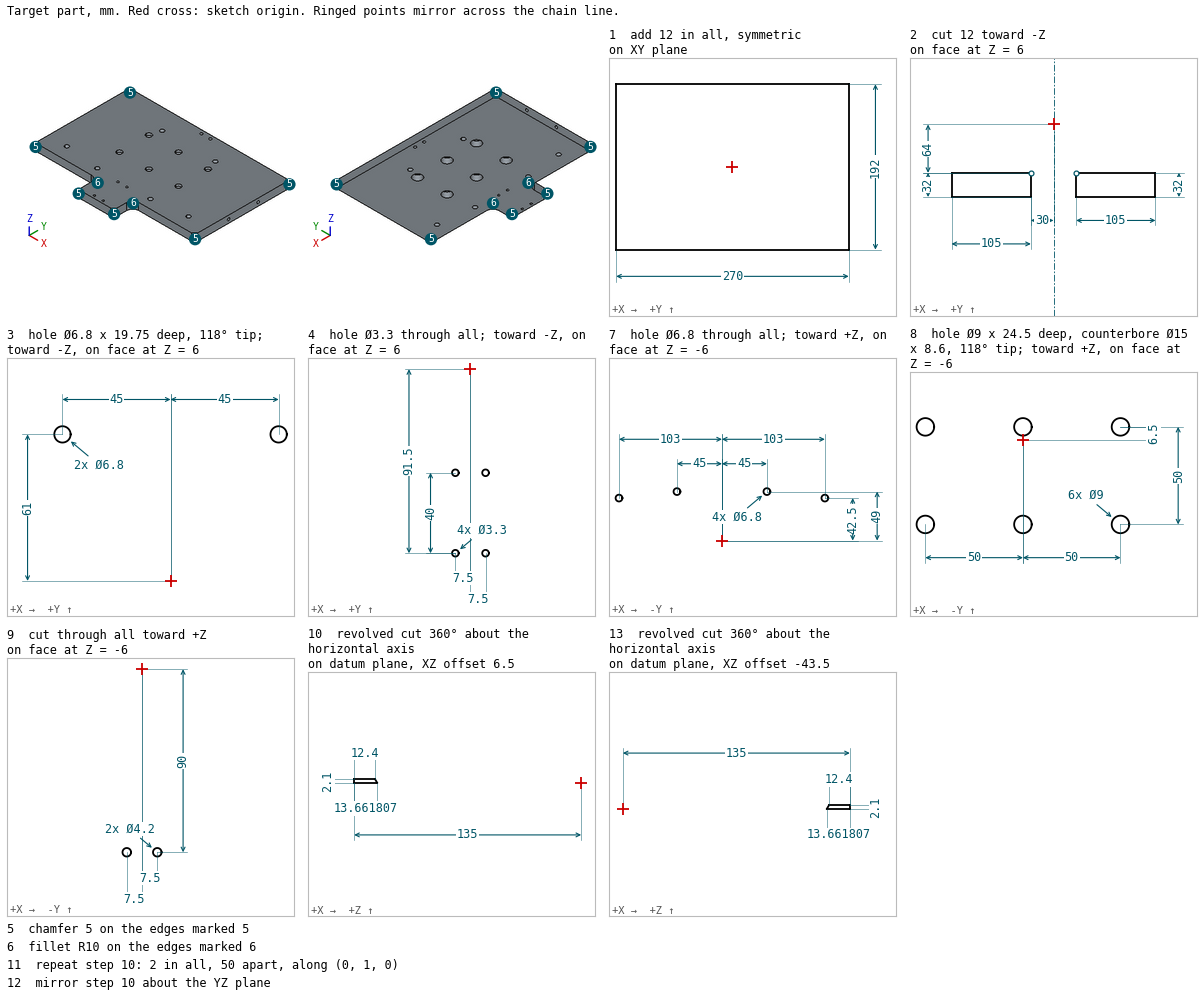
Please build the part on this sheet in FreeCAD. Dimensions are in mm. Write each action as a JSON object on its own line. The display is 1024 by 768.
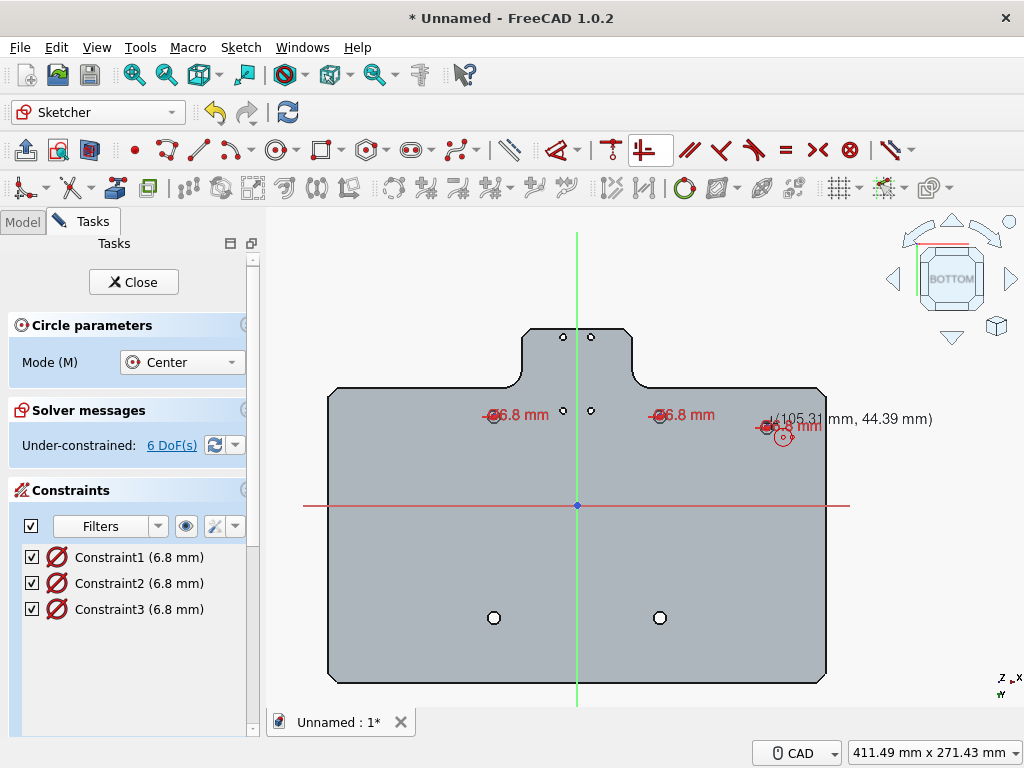
{"action": "scroll", "coordinate": [387, 427], "scroll_direction": "up", "scroll_amount": 7}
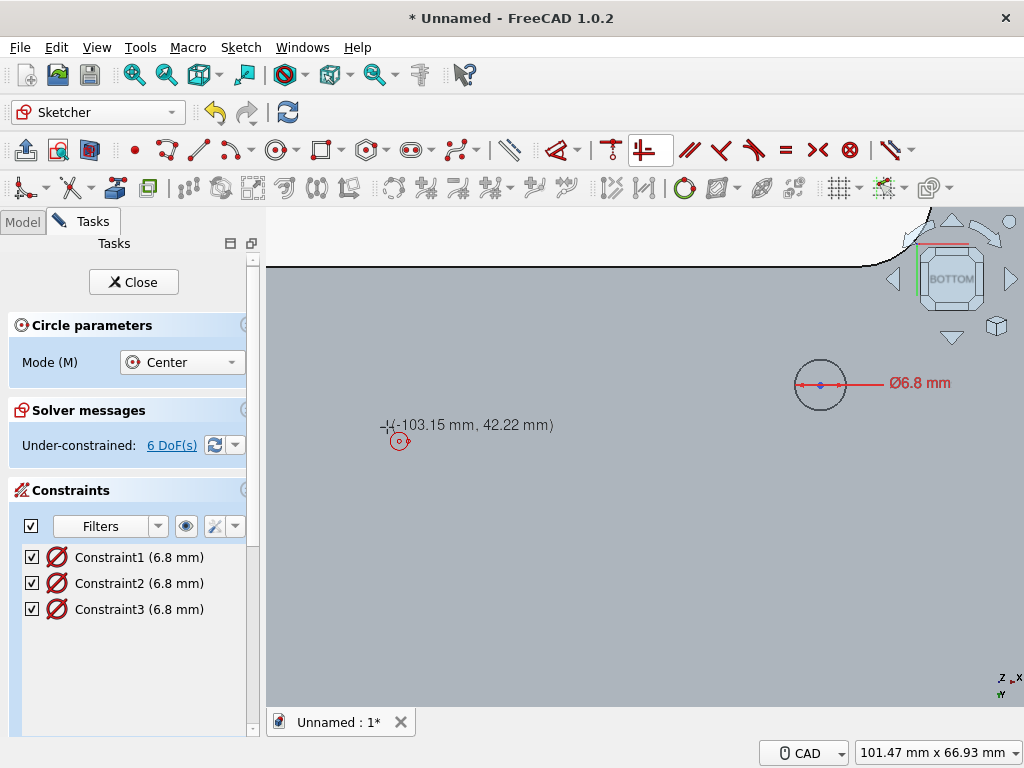
{"action": "scroll", "coordinate": [386, 427], "scroll_direction": "down", "scroll_amount": 7}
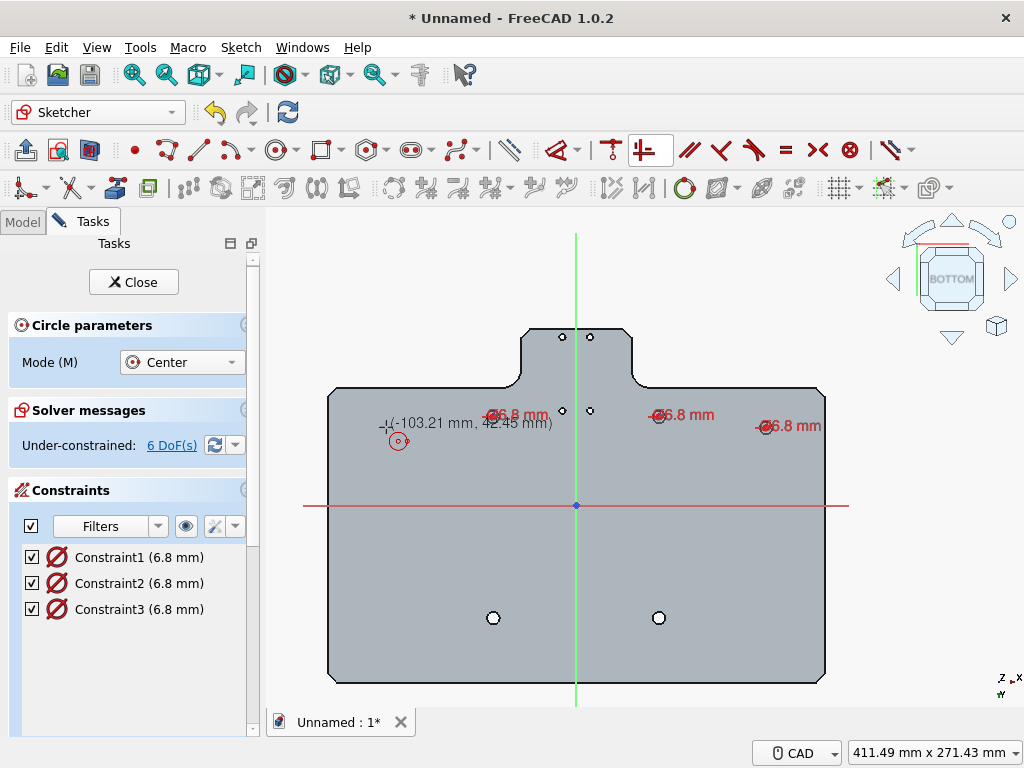
{"action": "left_click", "coordinate": [387, 427]}
{"action": "mouse_move", "coordinate": [391, 423]}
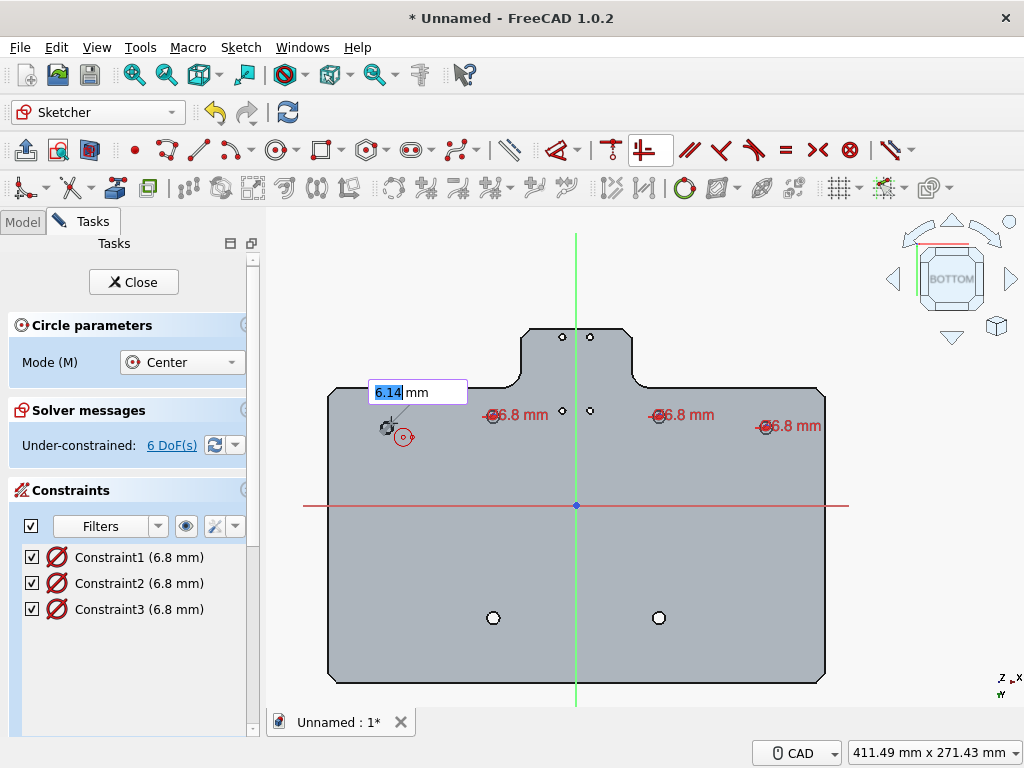
{"action": "type", "text": "6.8"}
{"action": "key", "text": "Return"}
{"action": "key", "text": "Escape"}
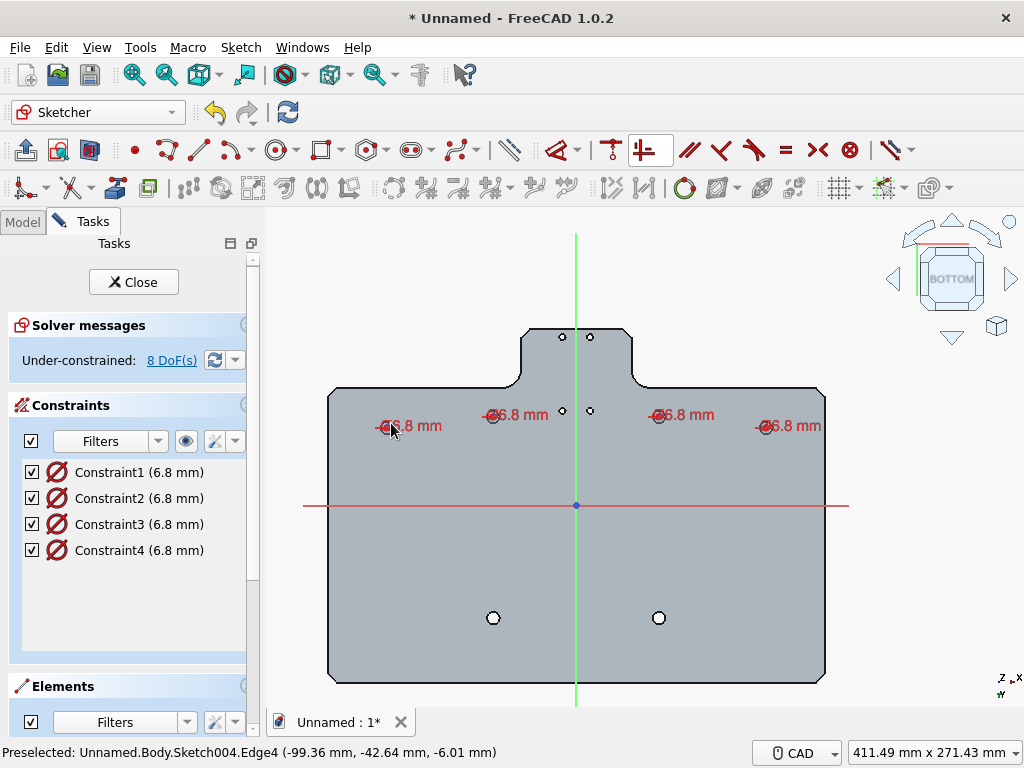
{"action": "left_click", "coordinate": [659, 417]}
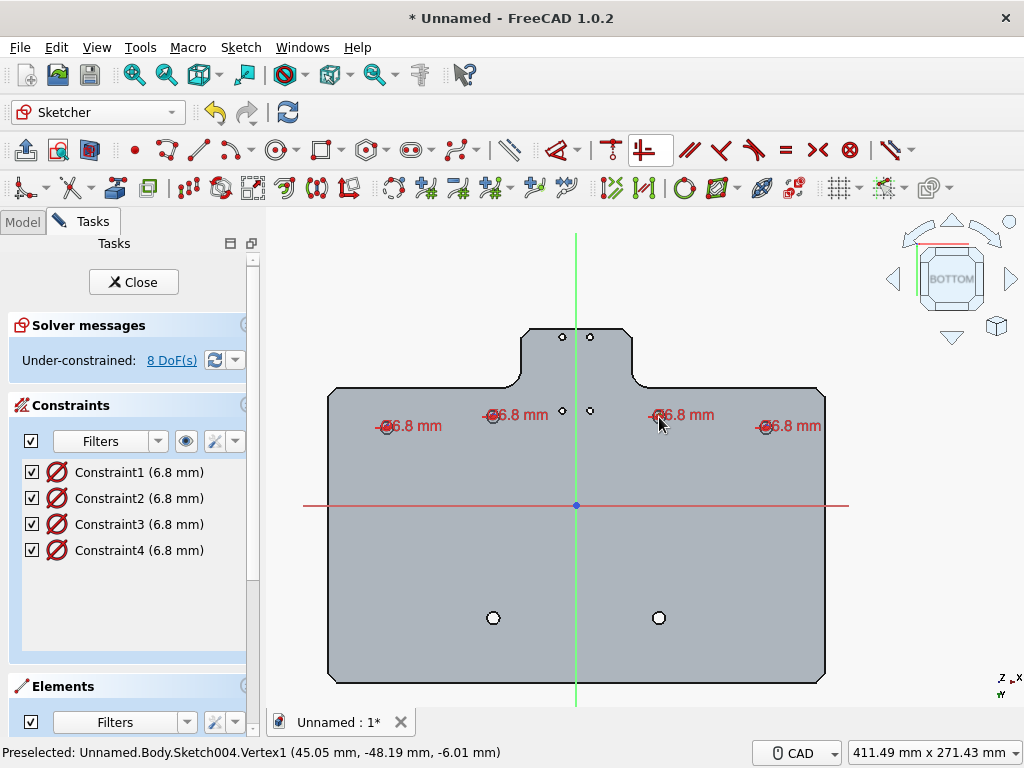
{"action": "left_click", "coordinate": [493, 417]}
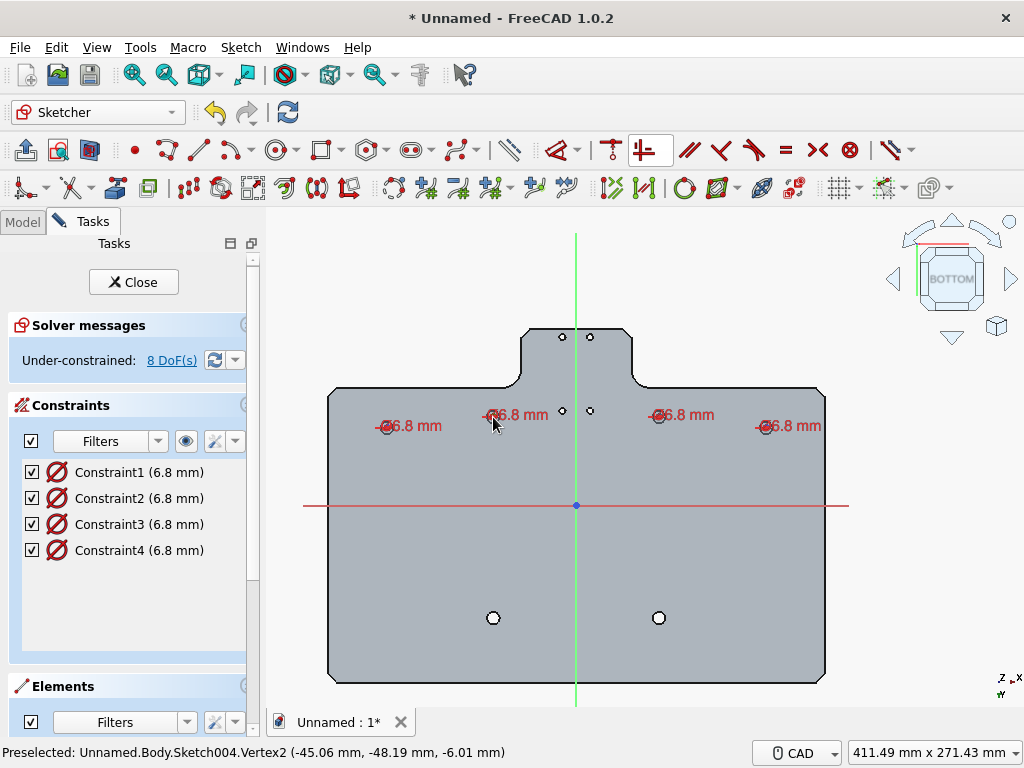
{"action": "key", "text": "h"}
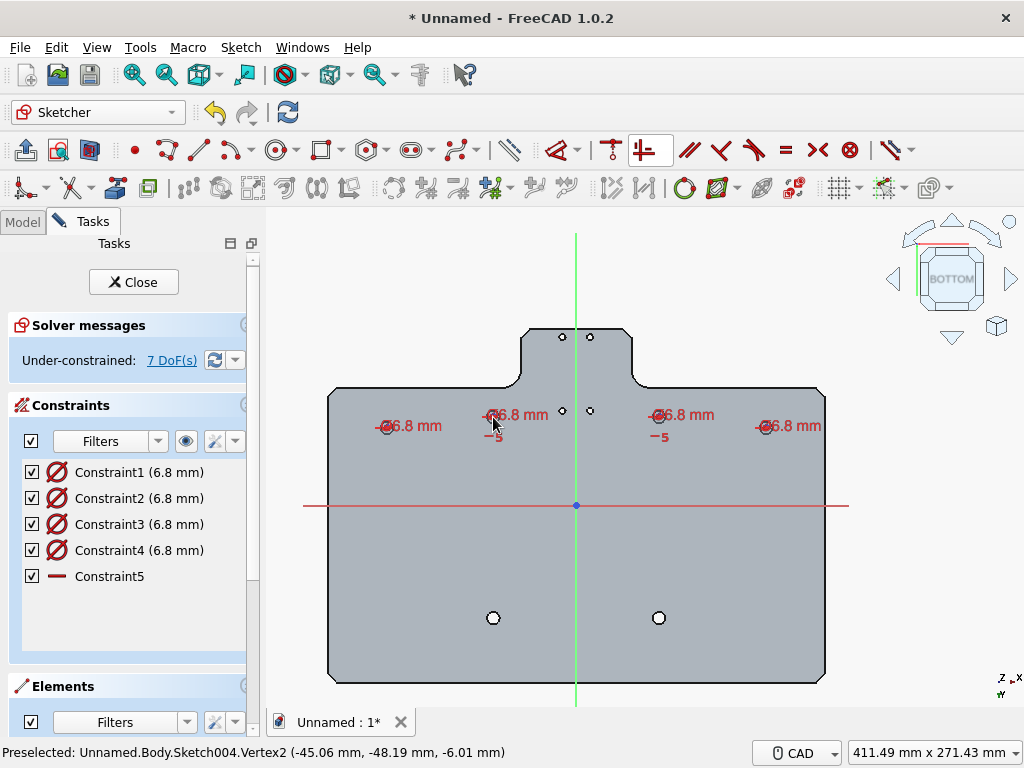
{"action": "left_click", "coordinate": [766, 428]}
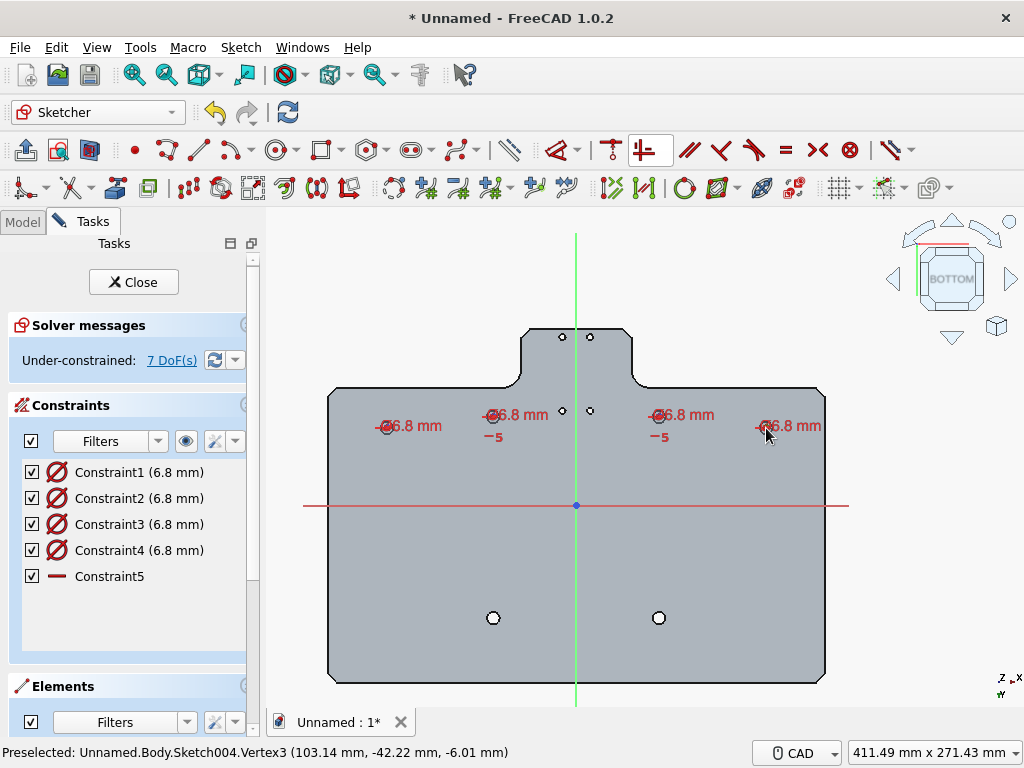
{"action": "left_click", "coordinate": [387, 428]}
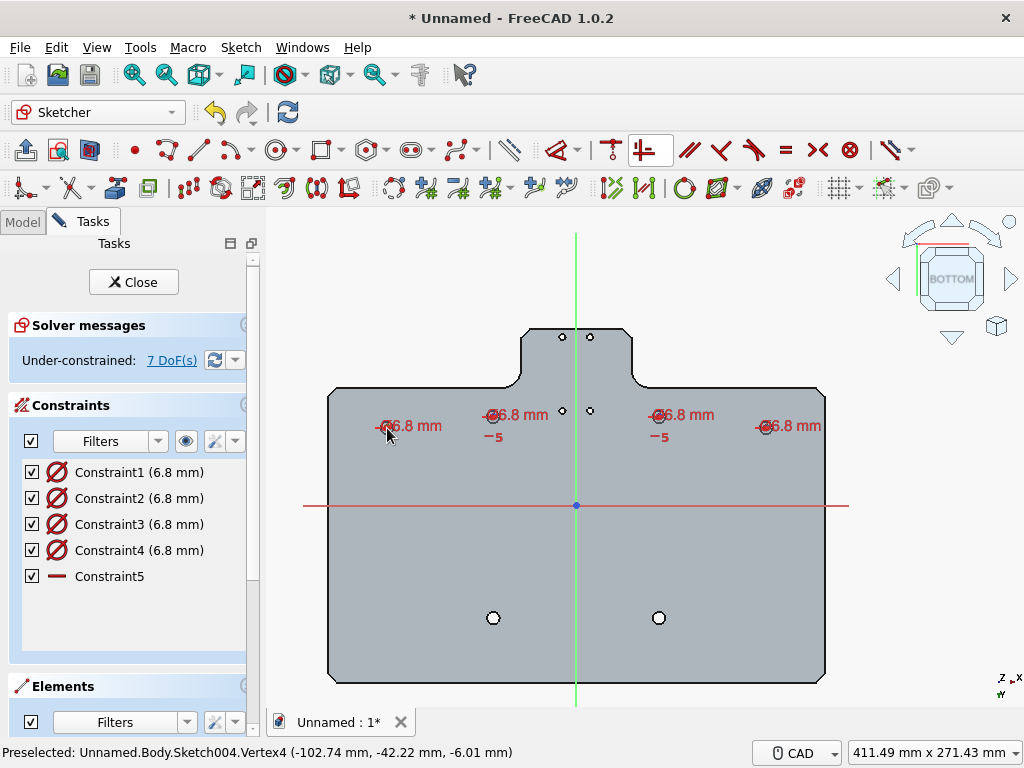
{"action": "key", "text": "h"}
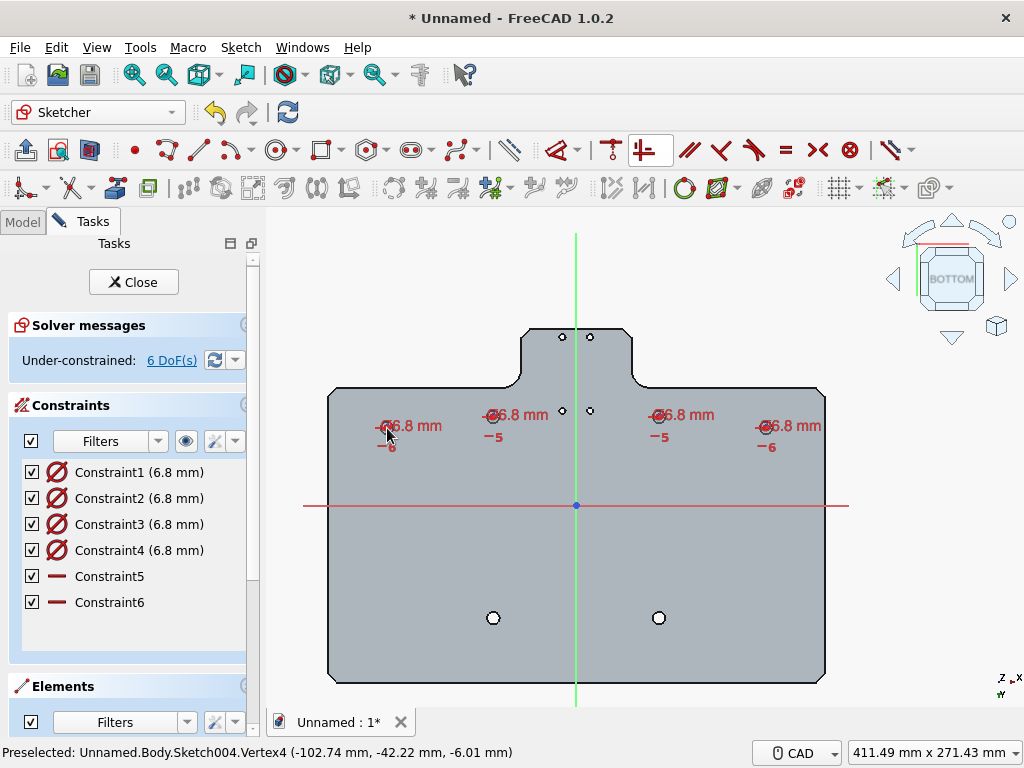
{"action": "left_click", "coordinate": [556, 150]}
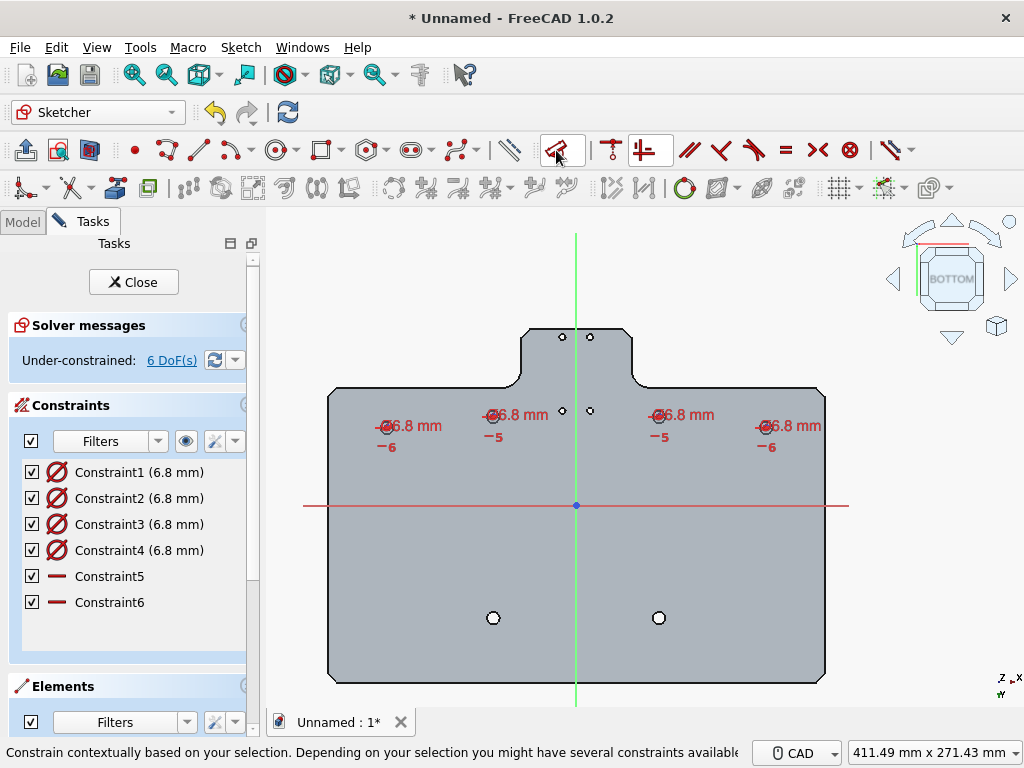
{"action": "left_click", "coordinate": [659, 417]}
{"action": "left_click", "coordinate": [618, 540]}